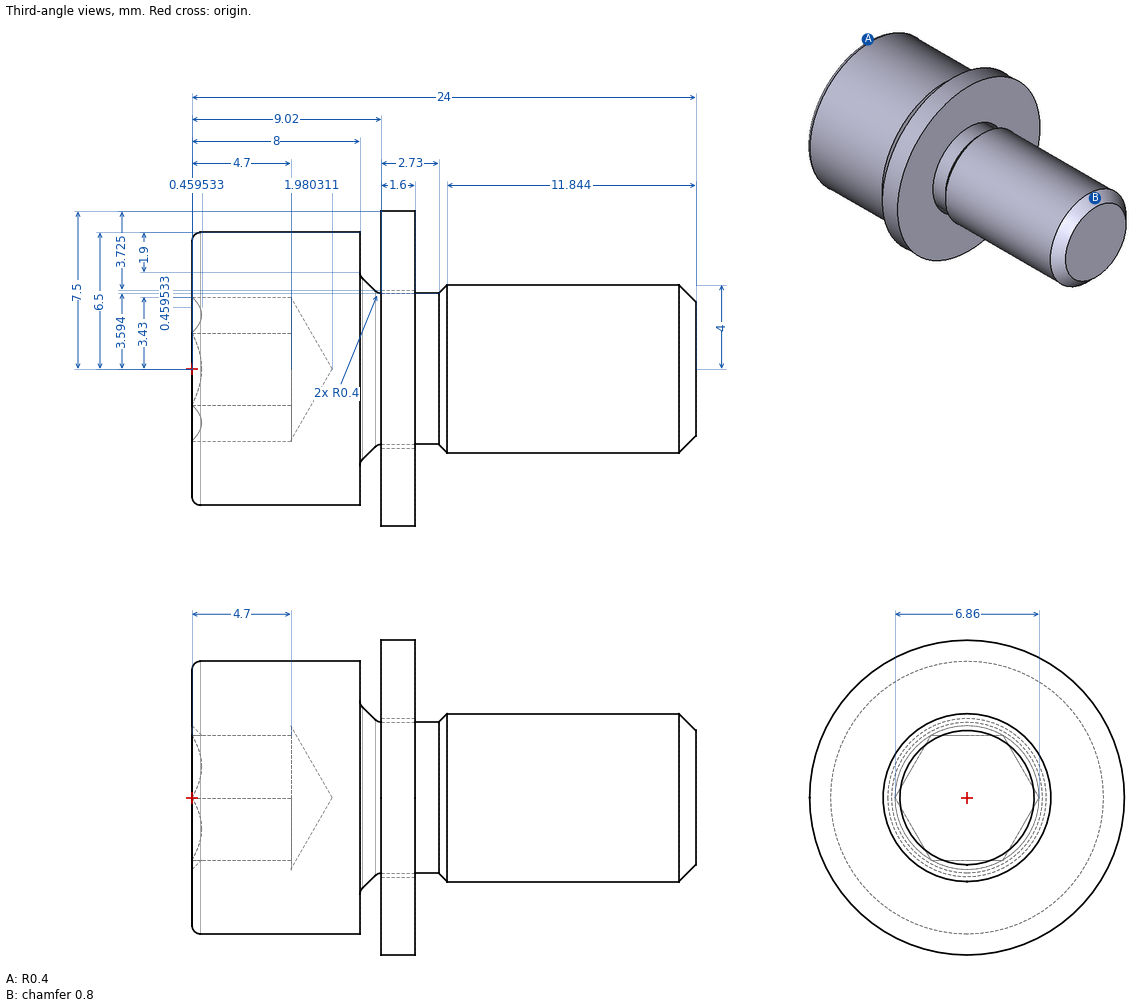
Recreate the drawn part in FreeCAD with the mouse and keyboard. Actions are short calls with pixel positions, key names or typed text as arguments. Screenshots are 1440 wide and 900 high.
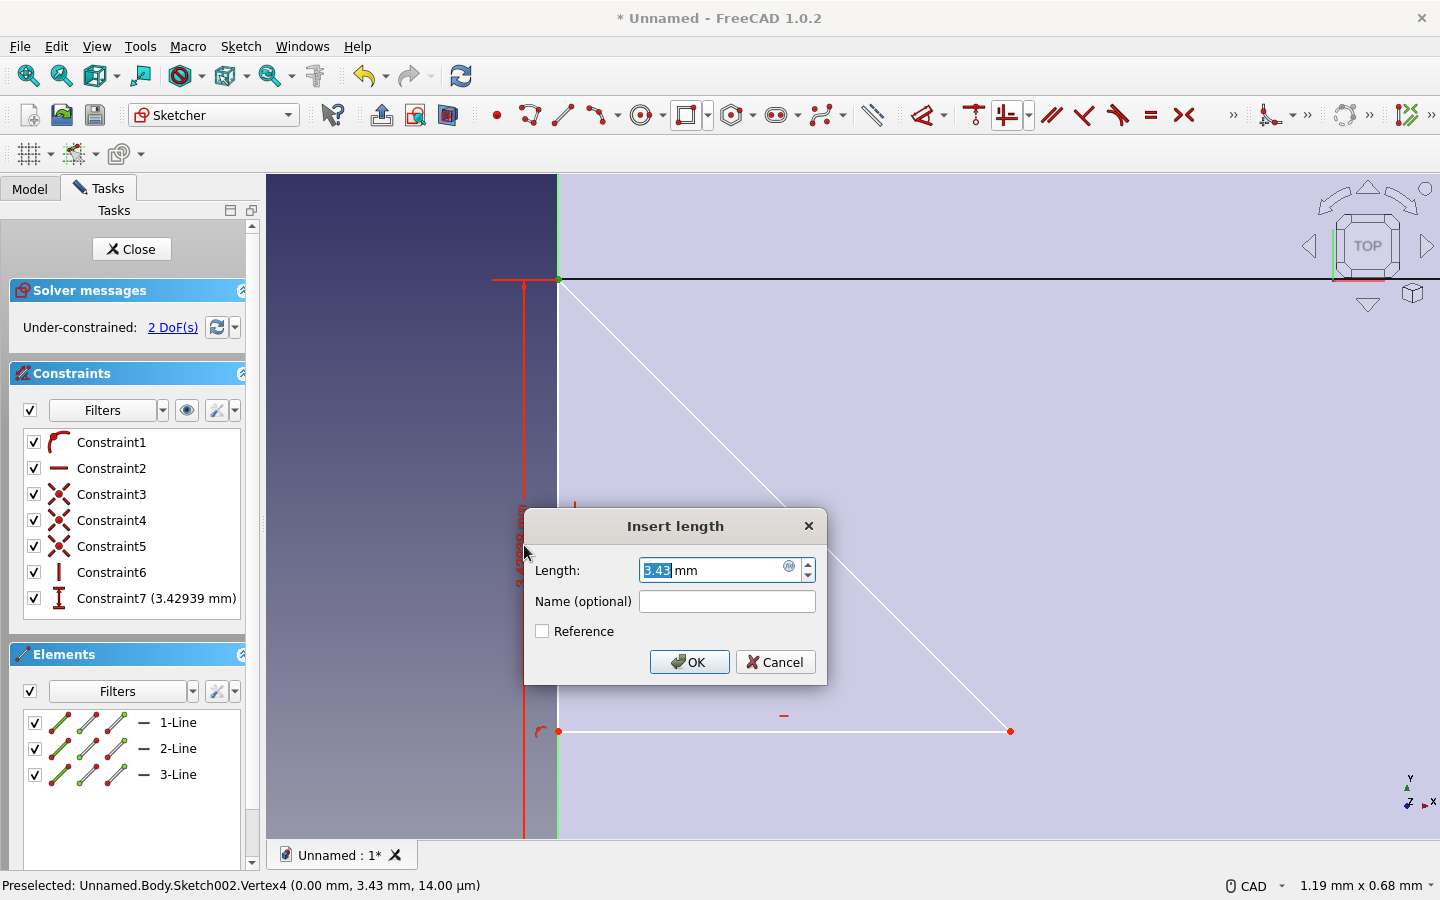
text(3.43)
key(Return)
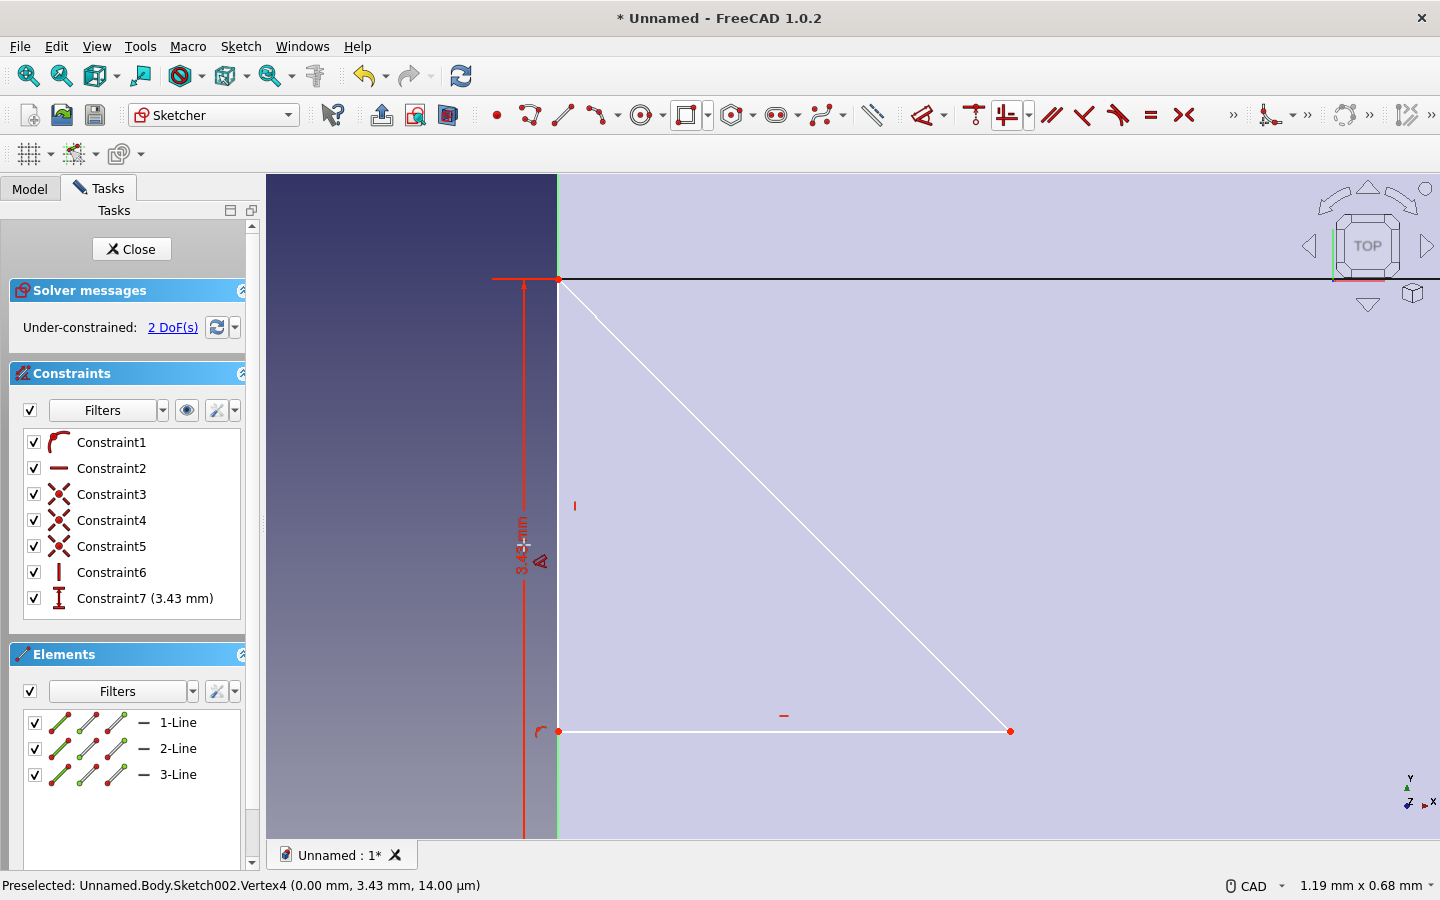
click(694, 732)
click(784, 766)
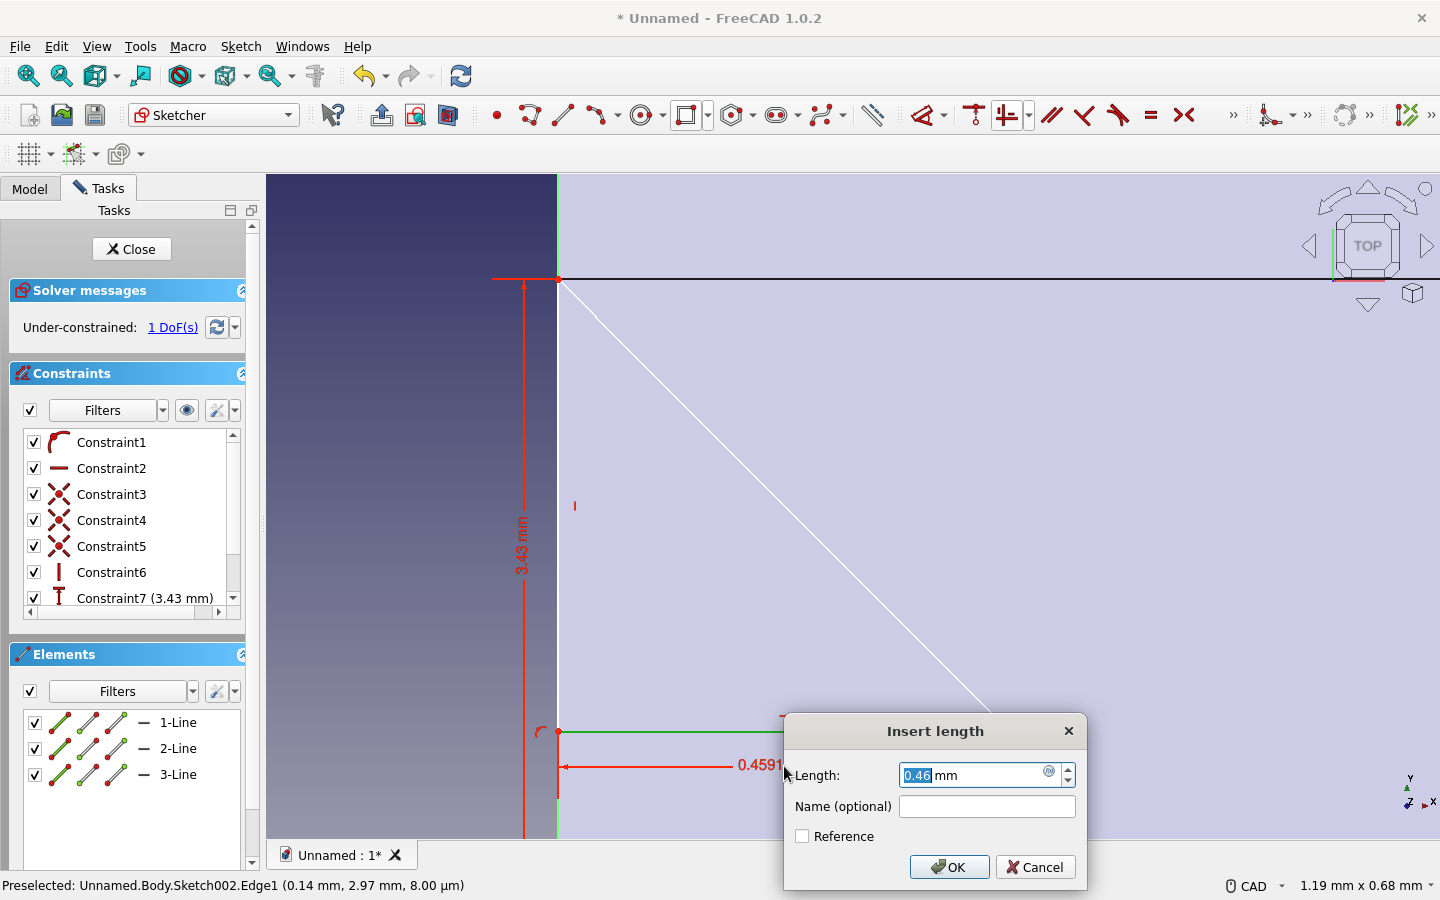
text(0.459533)
key(Return)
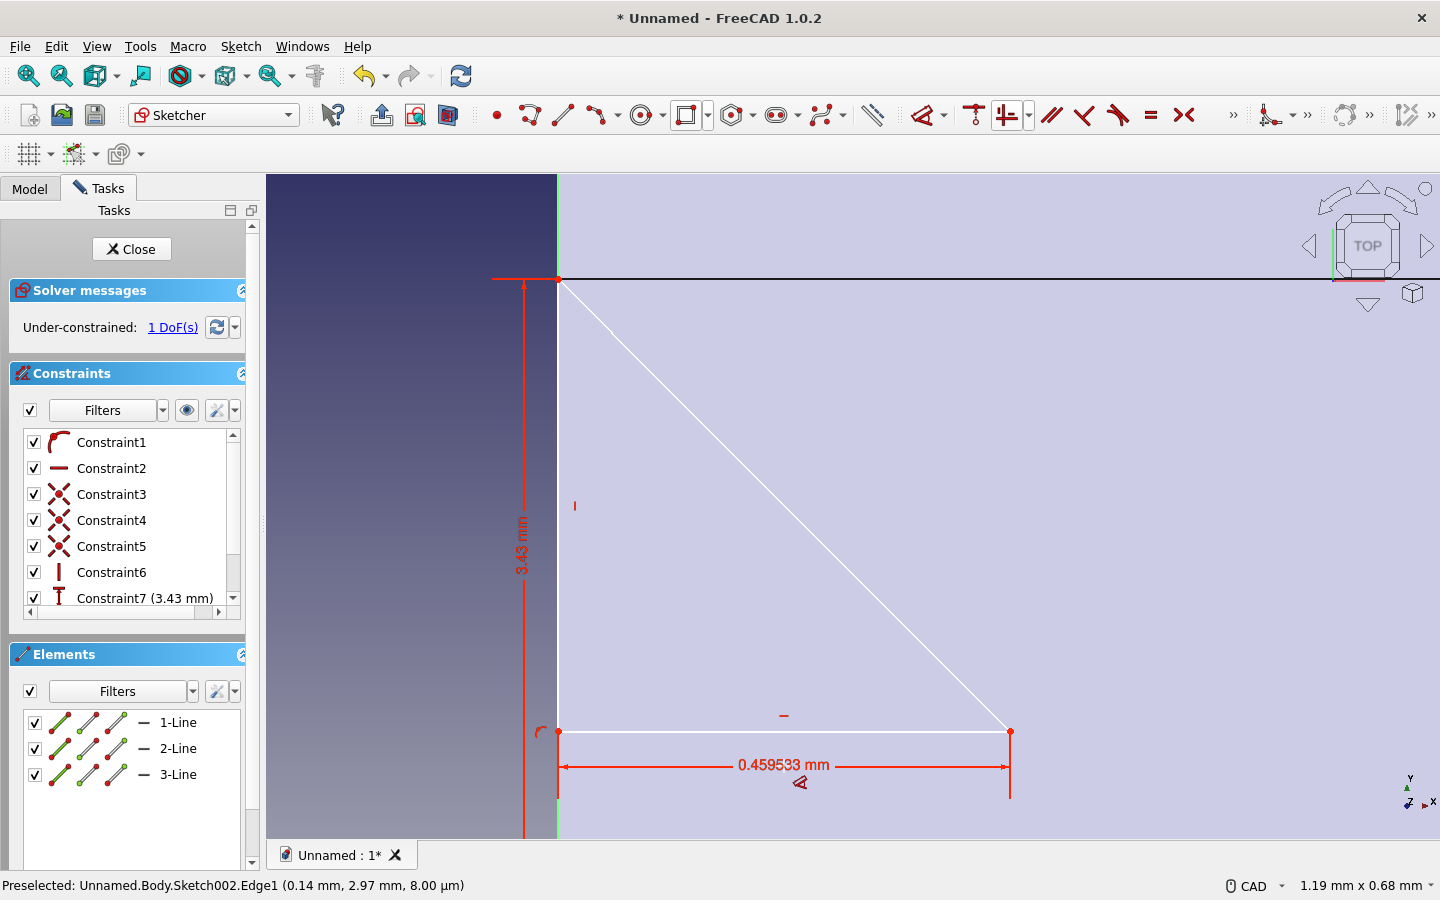
click(558, 415)
click(524, 506)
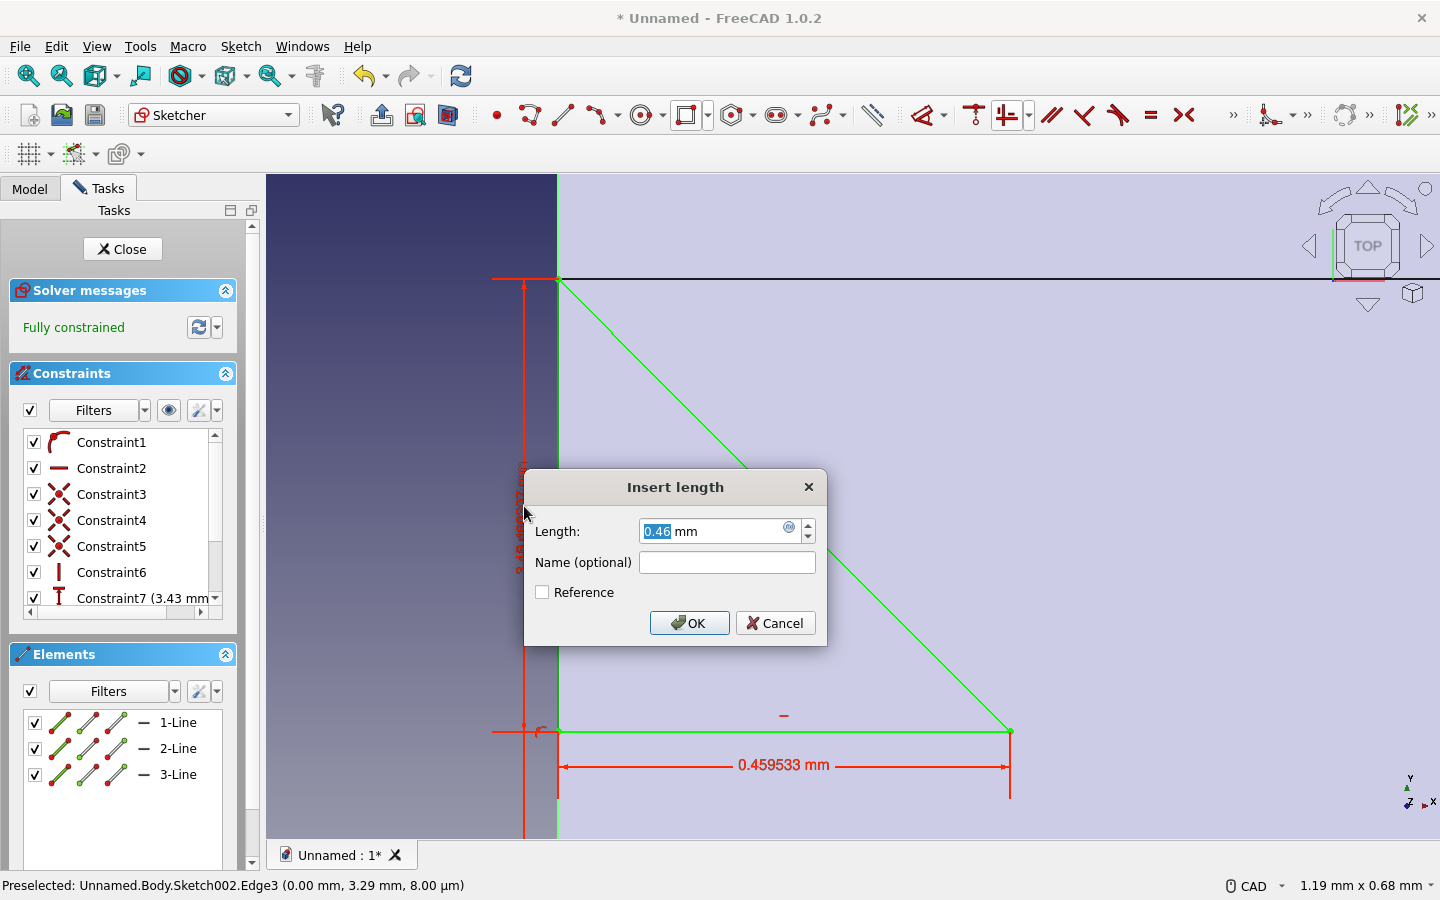
text(0.459533)
key(Return)
key(Escape)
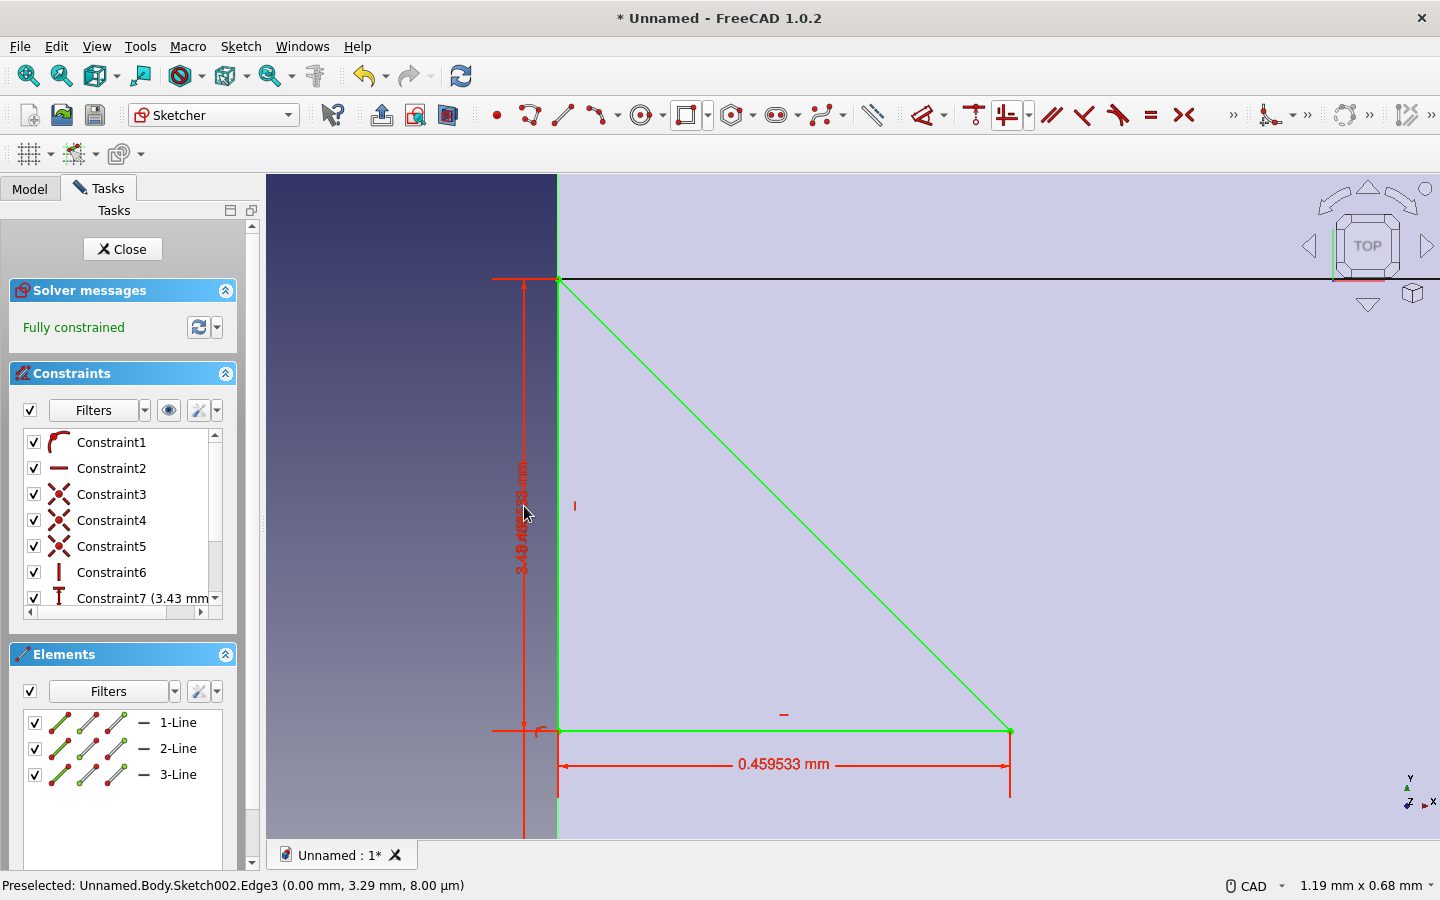
click(123, 249)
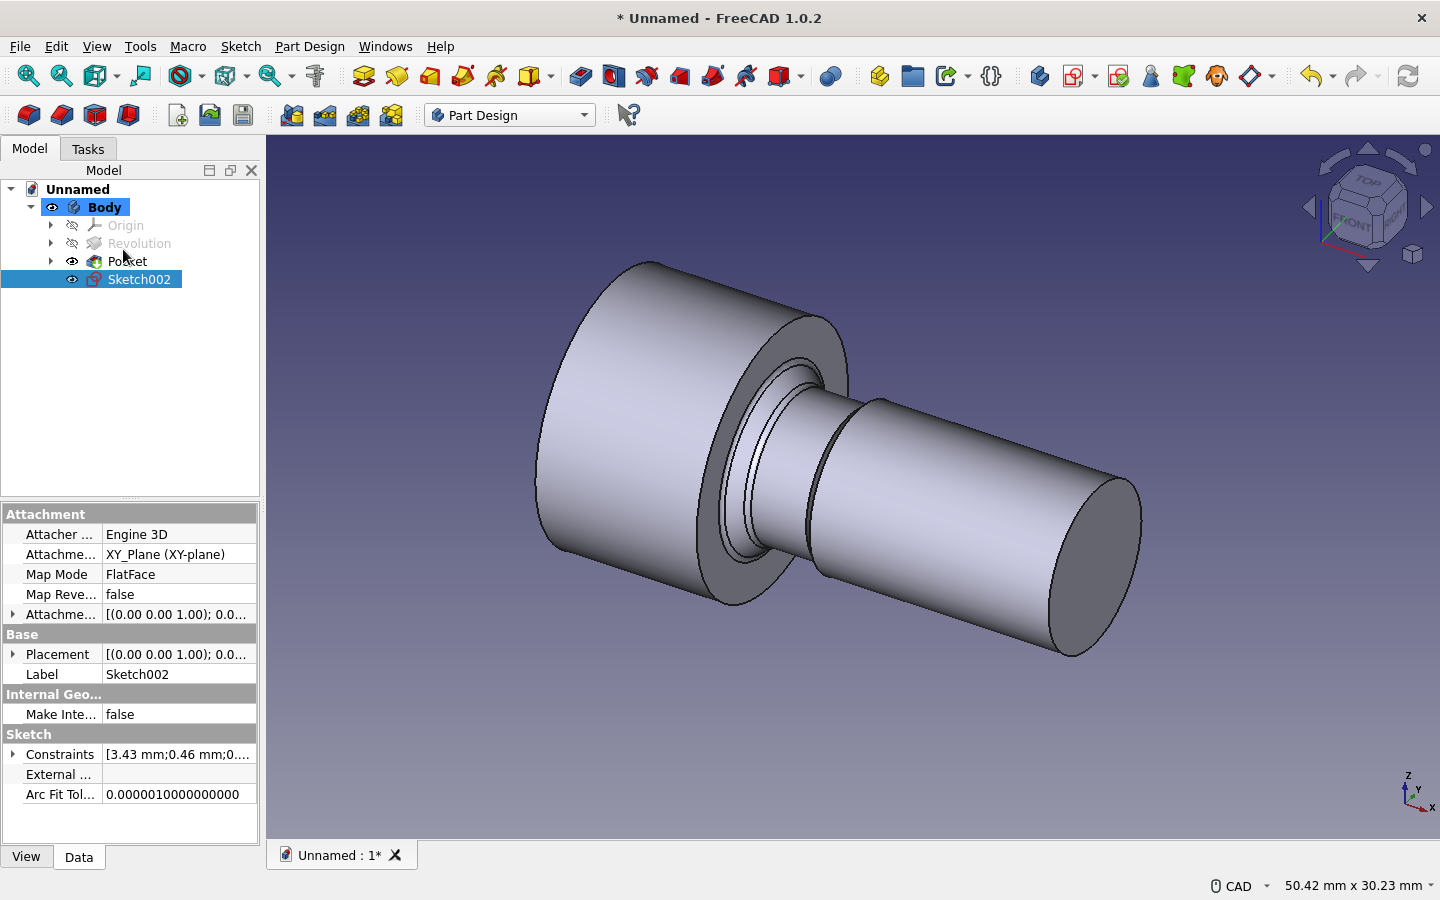
click(647, 76)